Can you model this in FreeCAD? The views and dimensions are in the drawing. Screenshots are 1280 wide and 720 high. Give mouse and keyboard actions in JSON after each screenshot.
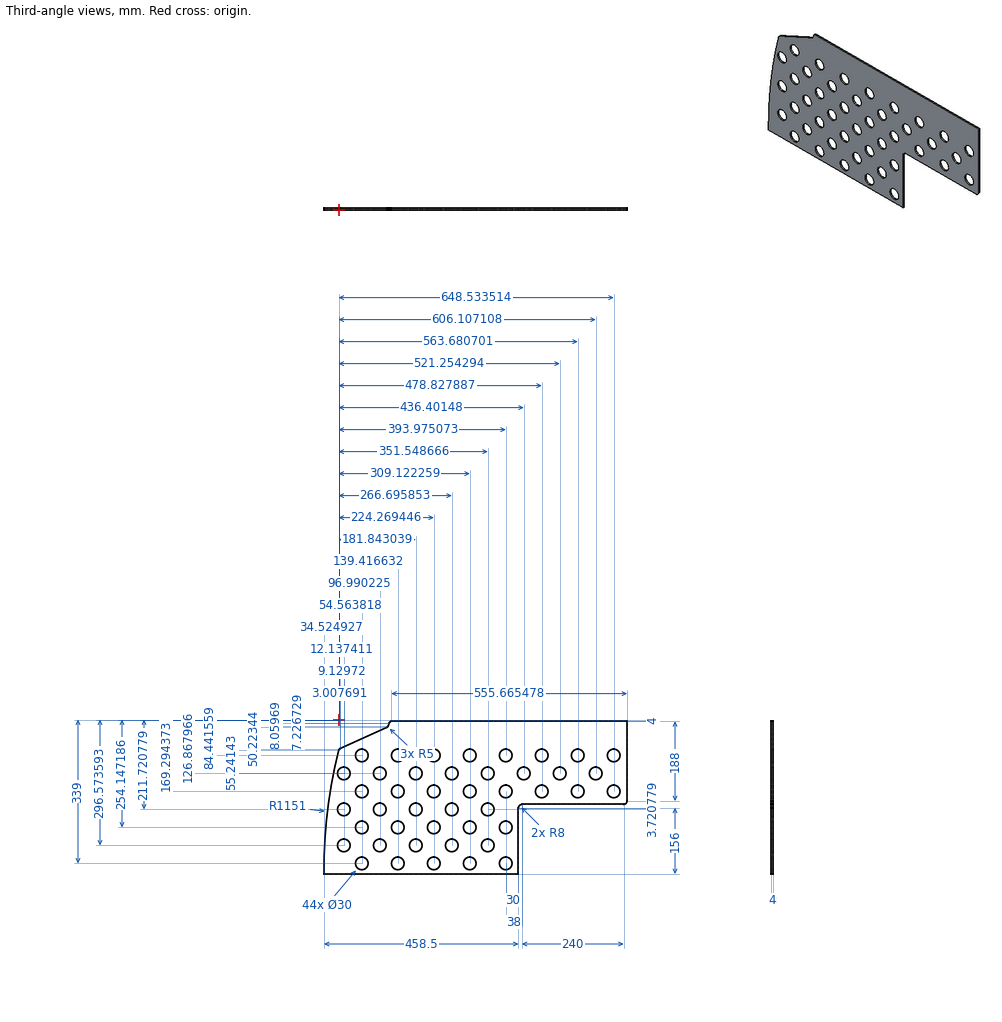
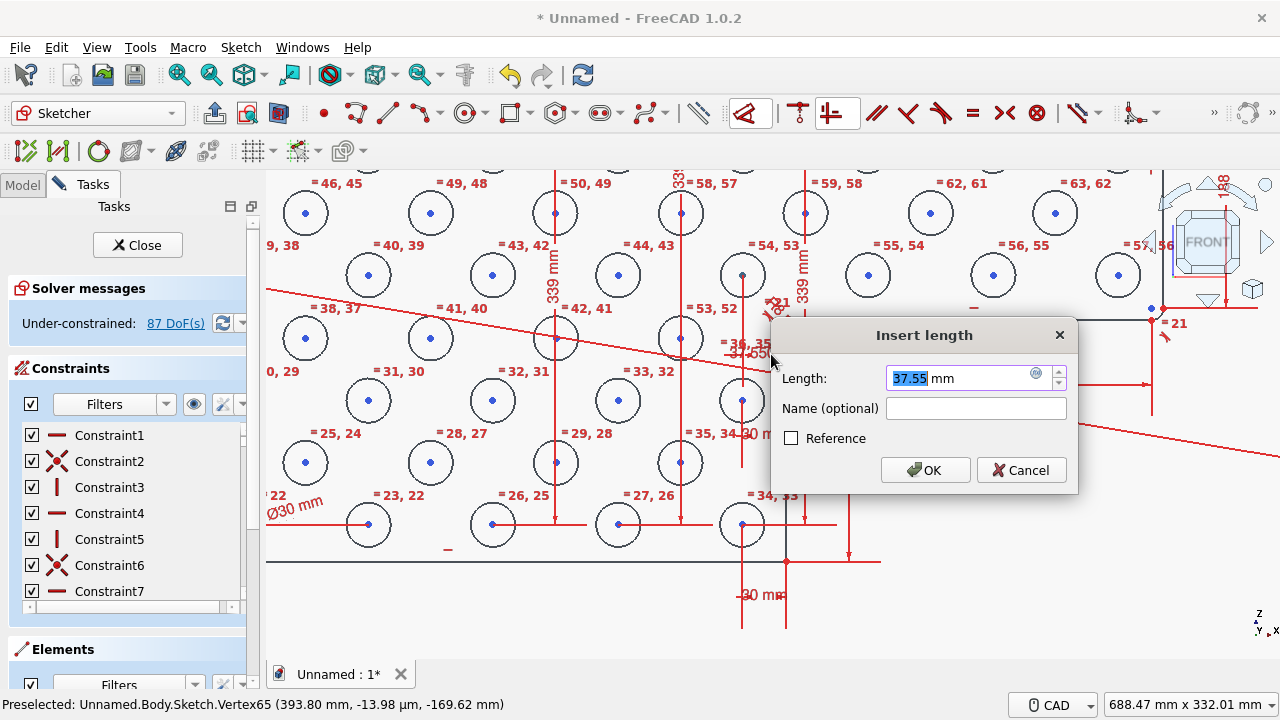
{"action": "type", "text": "38"}
{"action": "key", "text": "Return"}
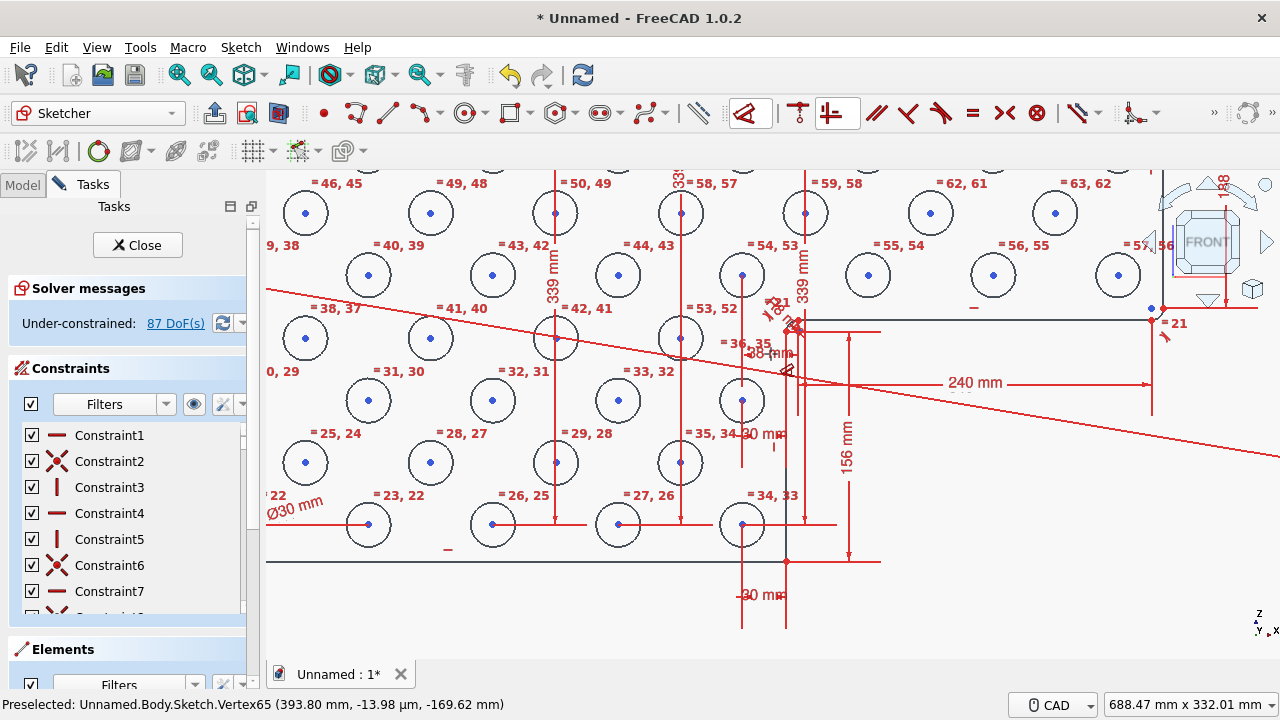
{"action": "left_click", "coordinate": [313, 562]}
{"action": "left_click", "coordinate": [540, 596]}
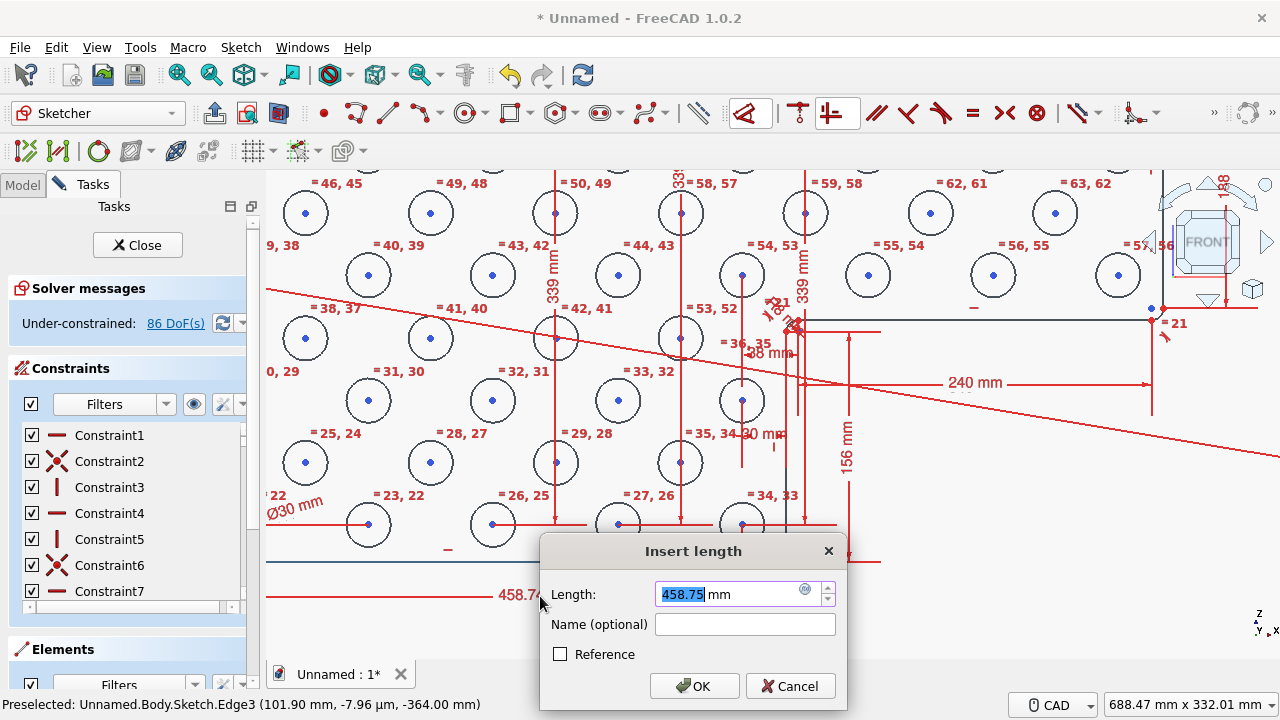
{"action": "type", "text": "458.5"}
{"action": "key", "text": "Return"}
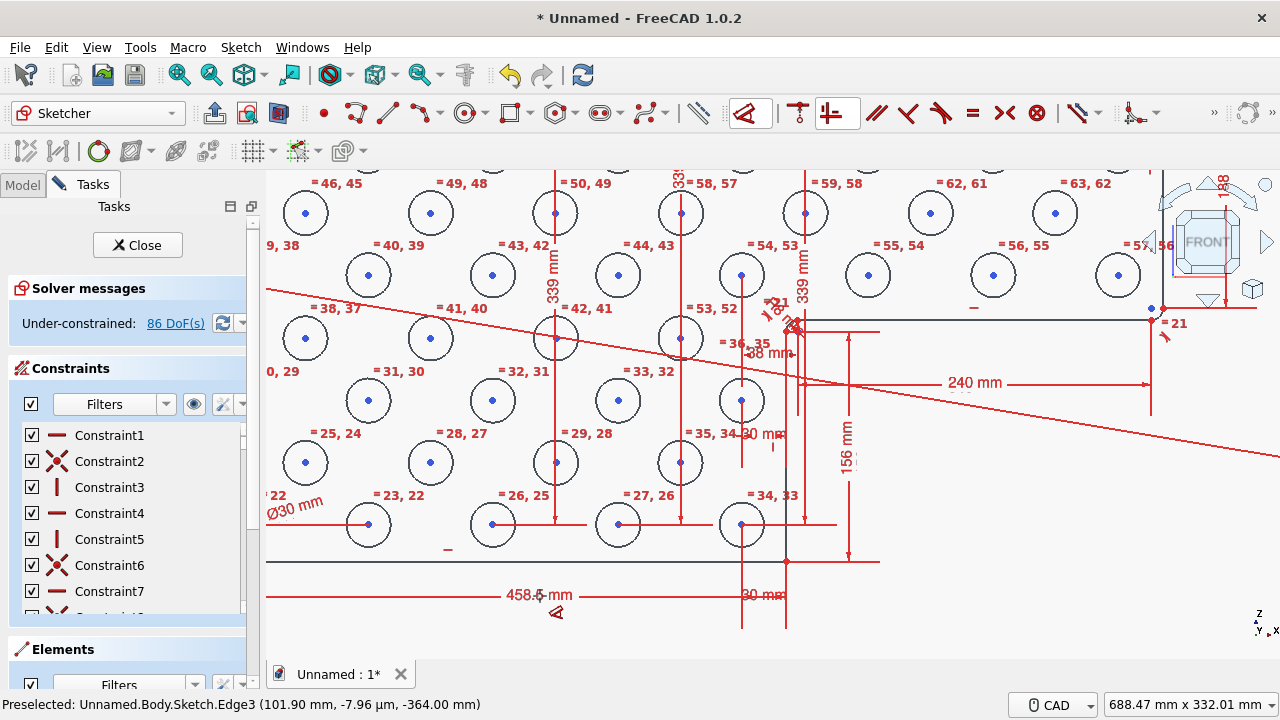
{"action": "scroll", "coordinate": [785, 562], "scroll_direction": "down", "scroll_amount": 3}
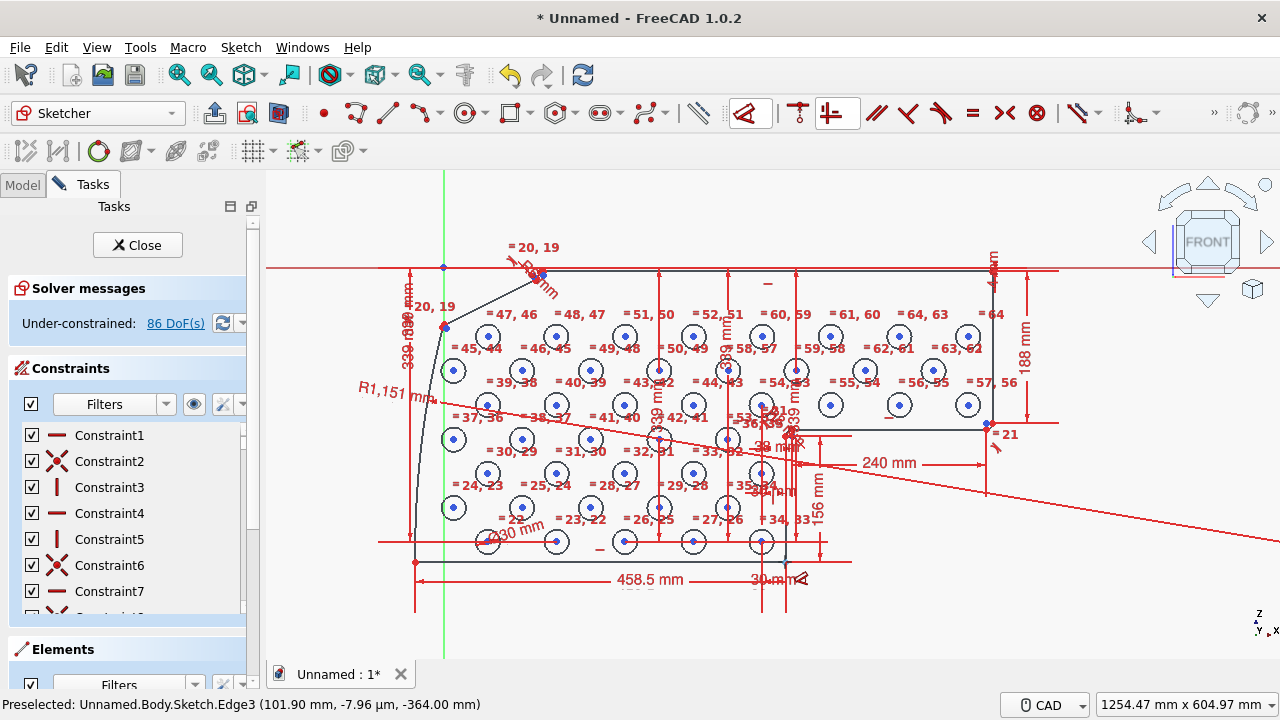
{"action": "scroll", "coordinate": [539, 276], "scroll_direction": "up", "scroll_amount": 10}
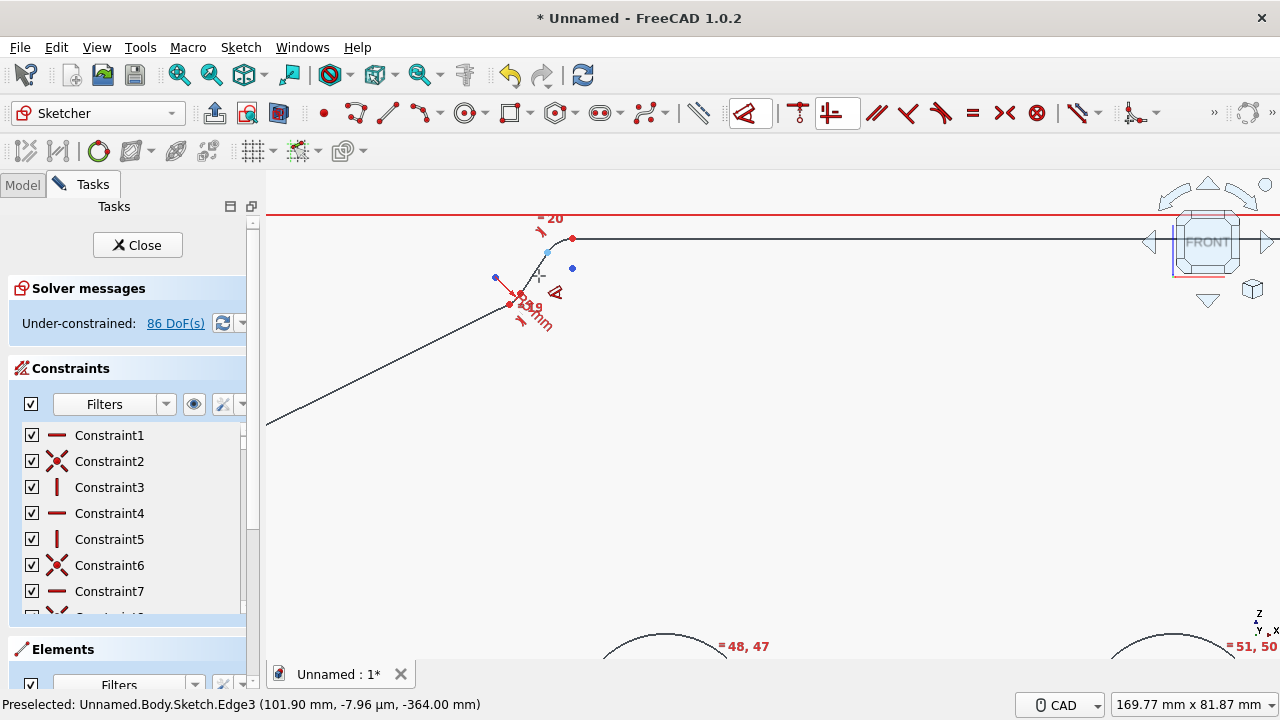
{"action": "left_click", "coordinate": [534, 273]}
{"action": "left_click", "coordinate": [487, 273]}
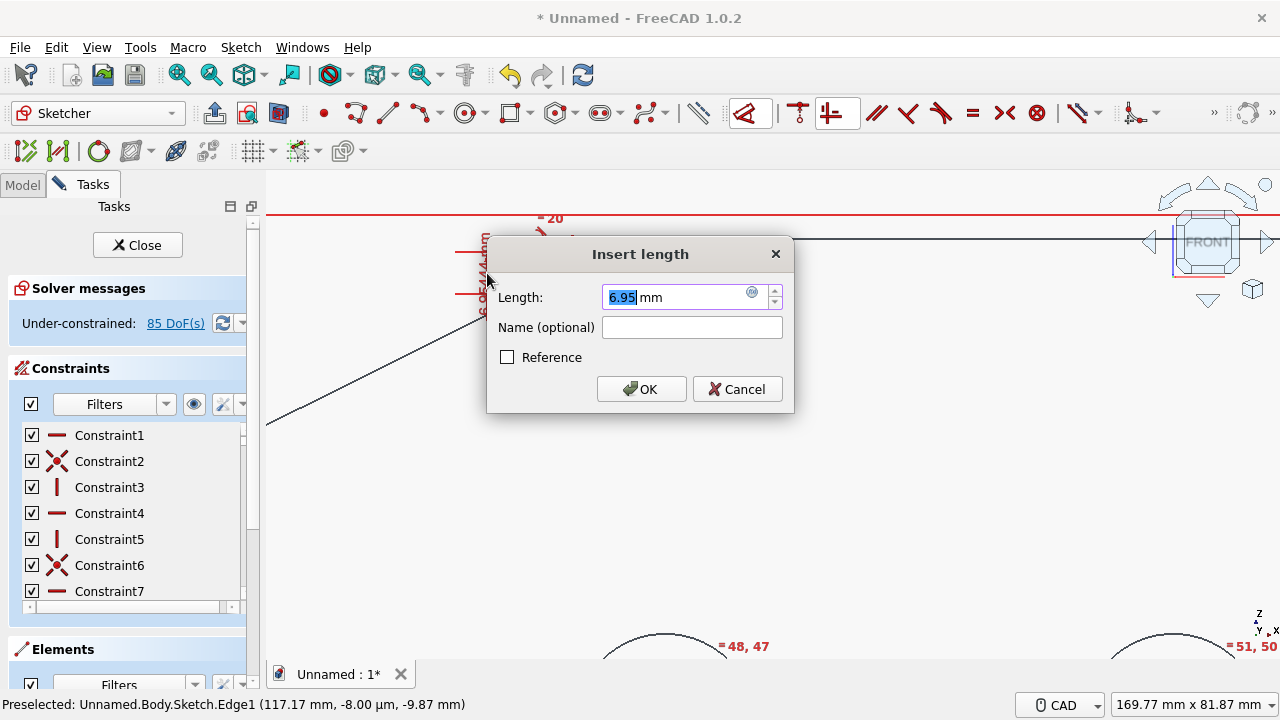
{"action": "type", "text": "8.05969"}
{"action": "key", "text": "Return"}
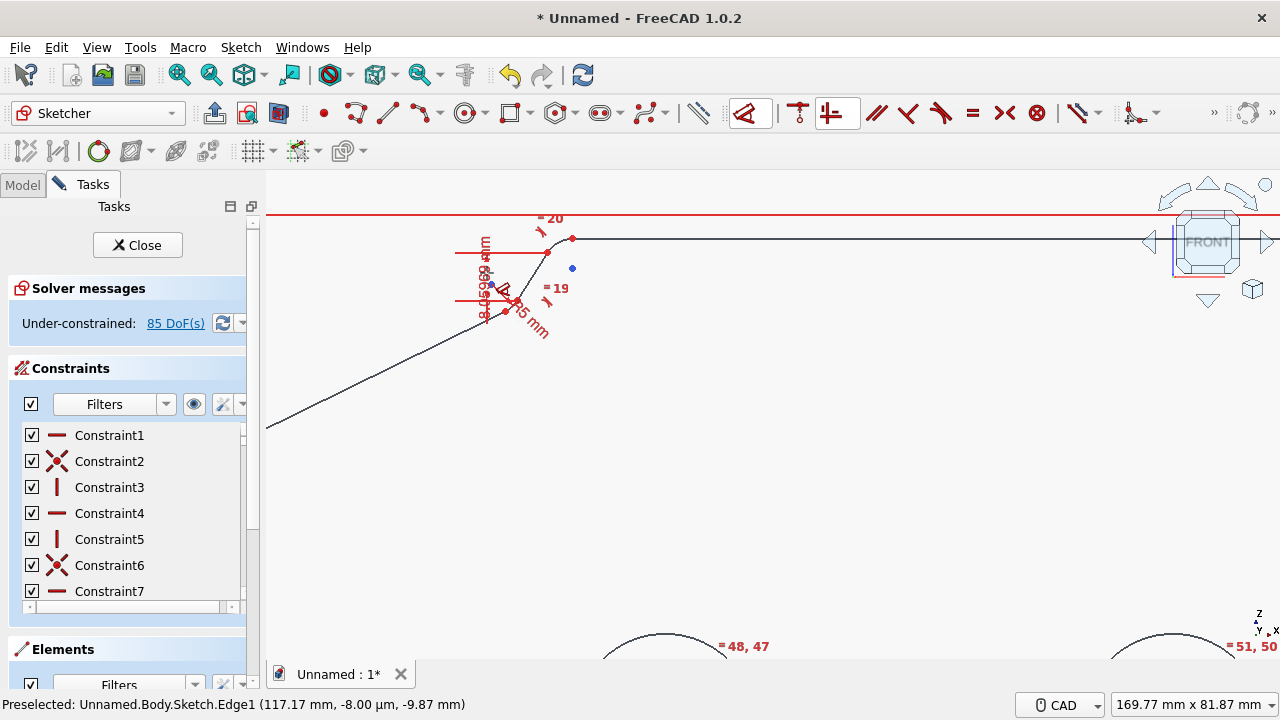
{"action": "scroll", "coordinate": [539, 276], "scroll_direction": "down", "scroll_amount": 10}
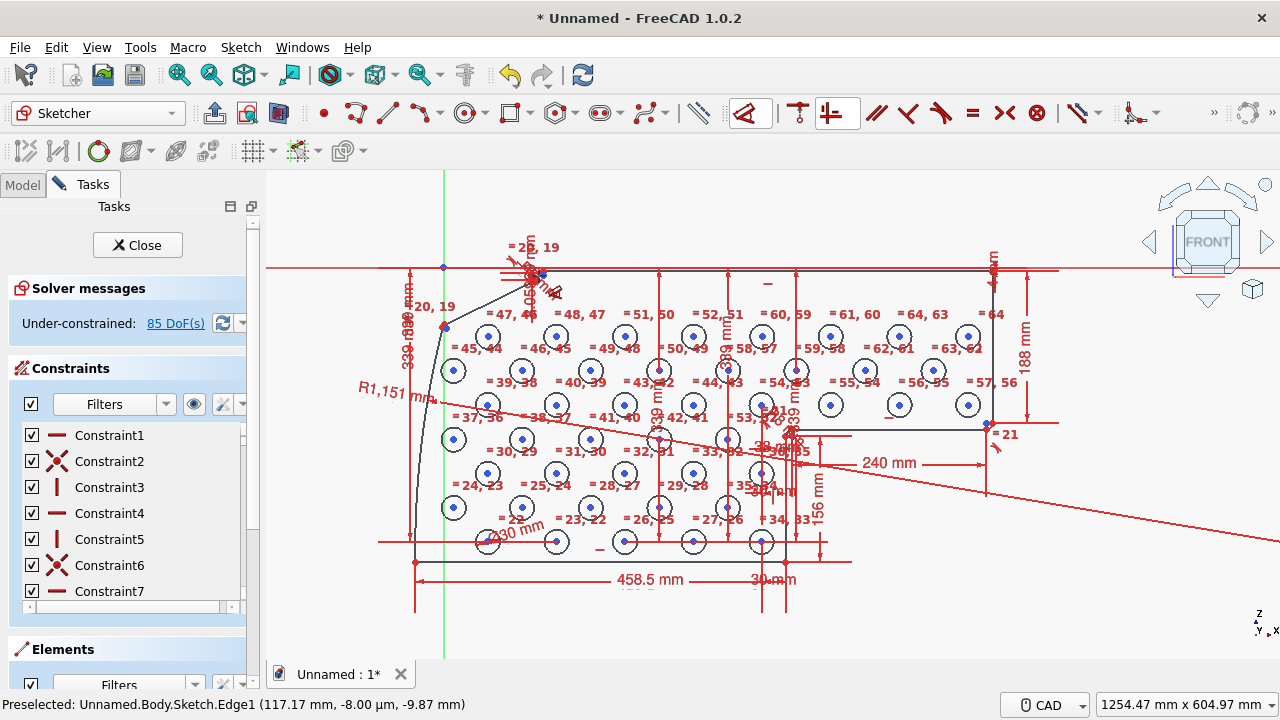
{"action": "scroll", "coordinate": [445, 325], "scroll_direction": "up", "scroll_amount": 9}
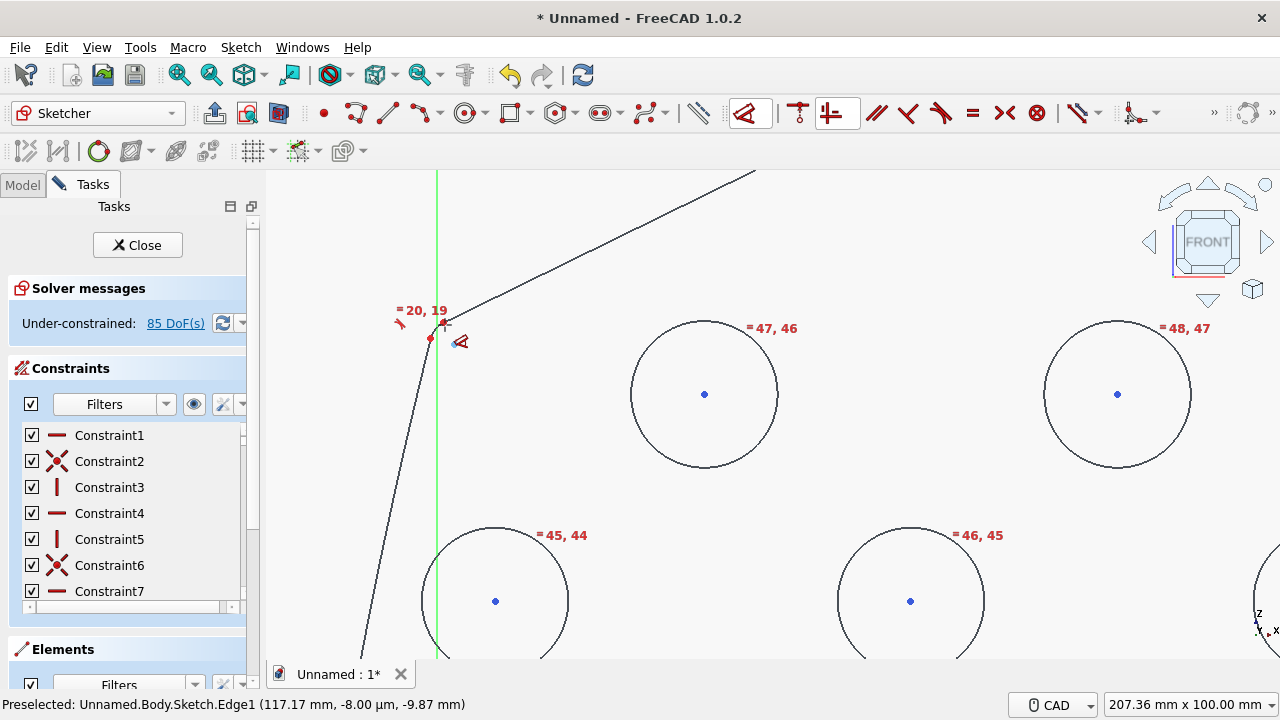
{"action": "left_click", "coordinate": [444, 323]}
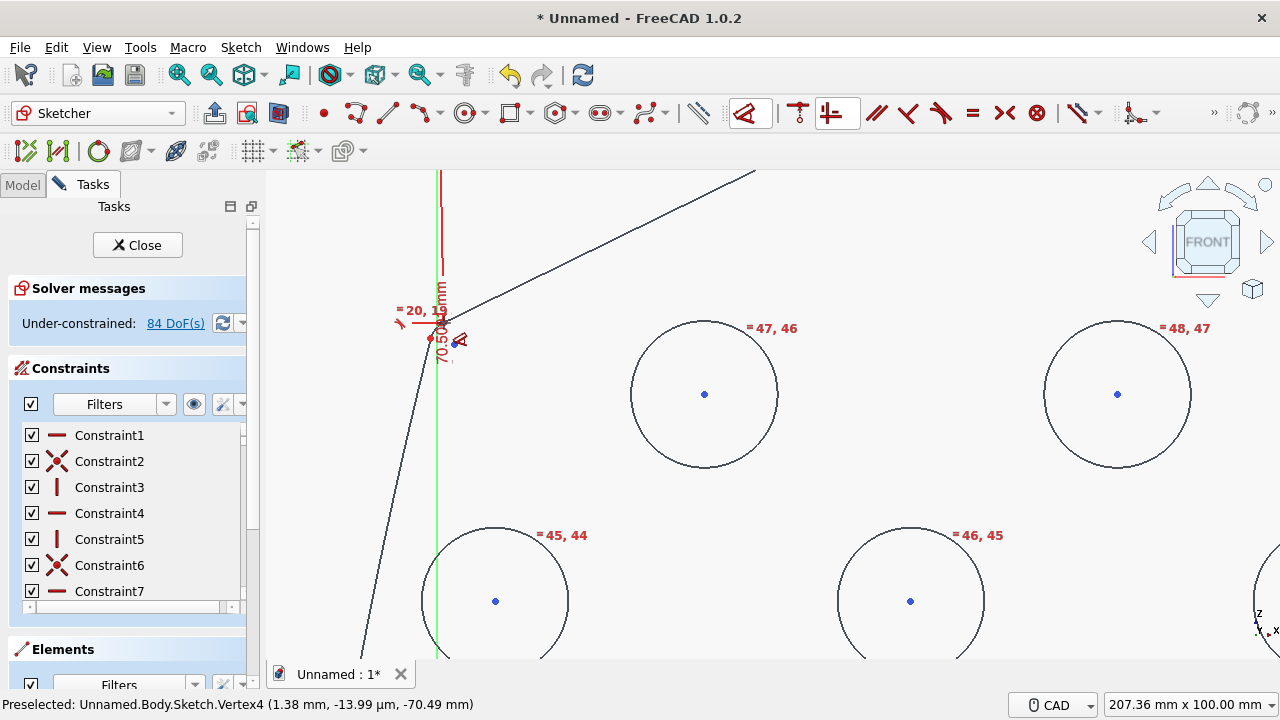
{"action": "left_click", "coordinate": [495, 601]}
{"action": "left_click", "coordinate": [469, 289]}